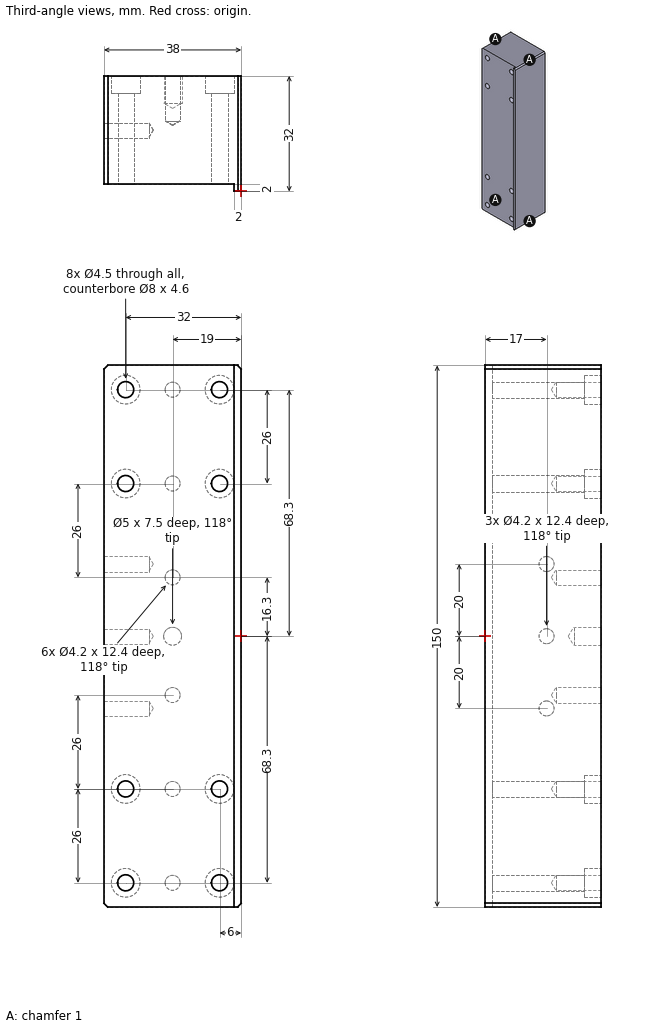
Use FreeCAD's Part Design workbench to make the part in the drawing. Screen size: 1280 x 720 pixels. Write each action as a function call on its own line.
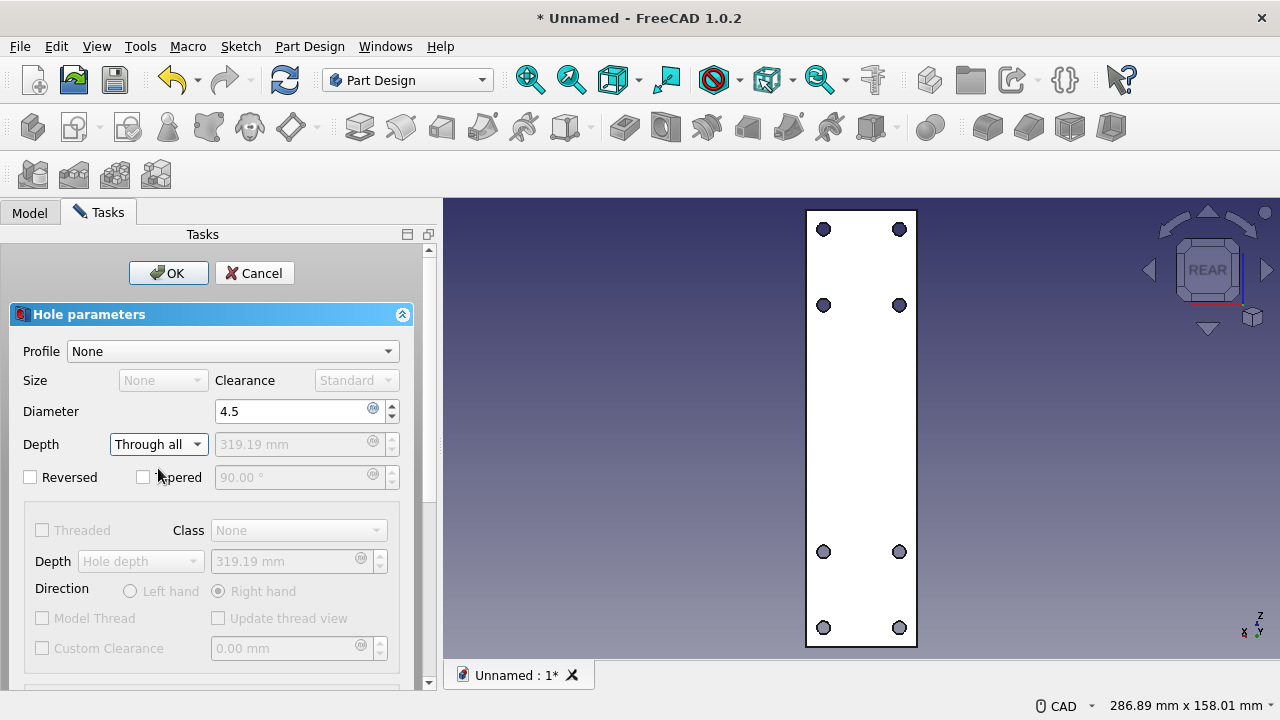
scroll(429, 467, down, 2)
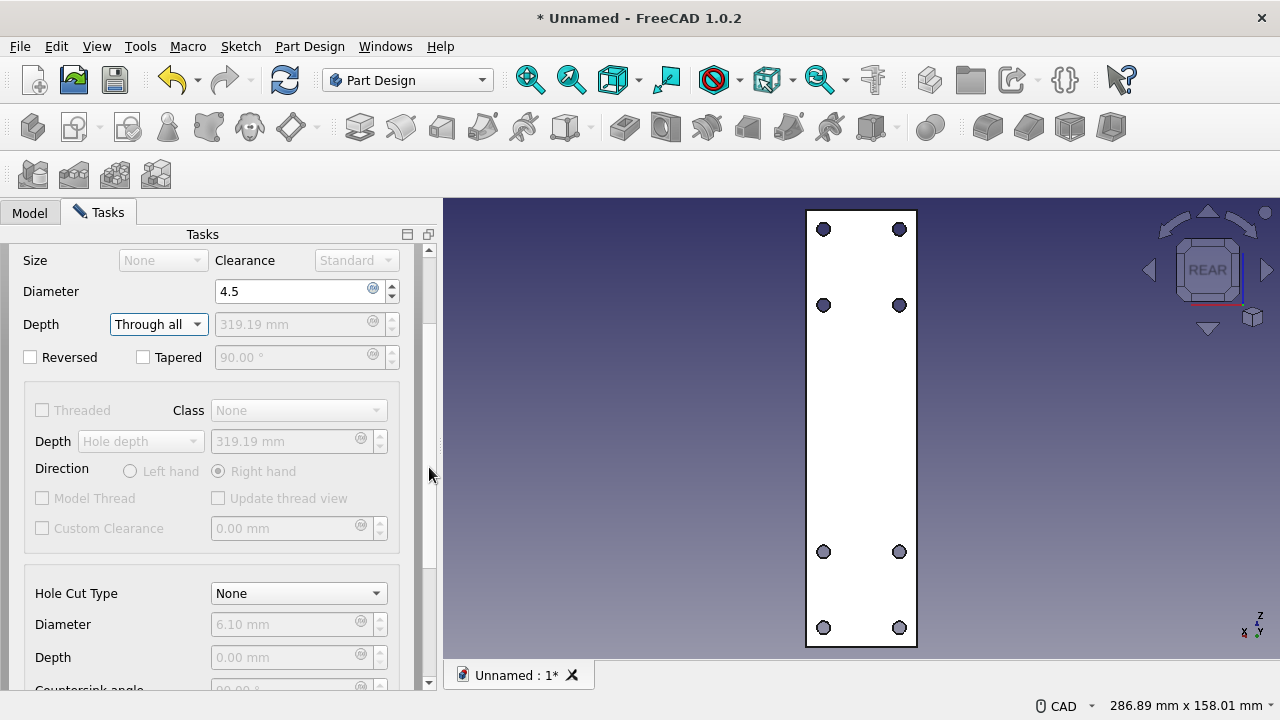
click(300, 594)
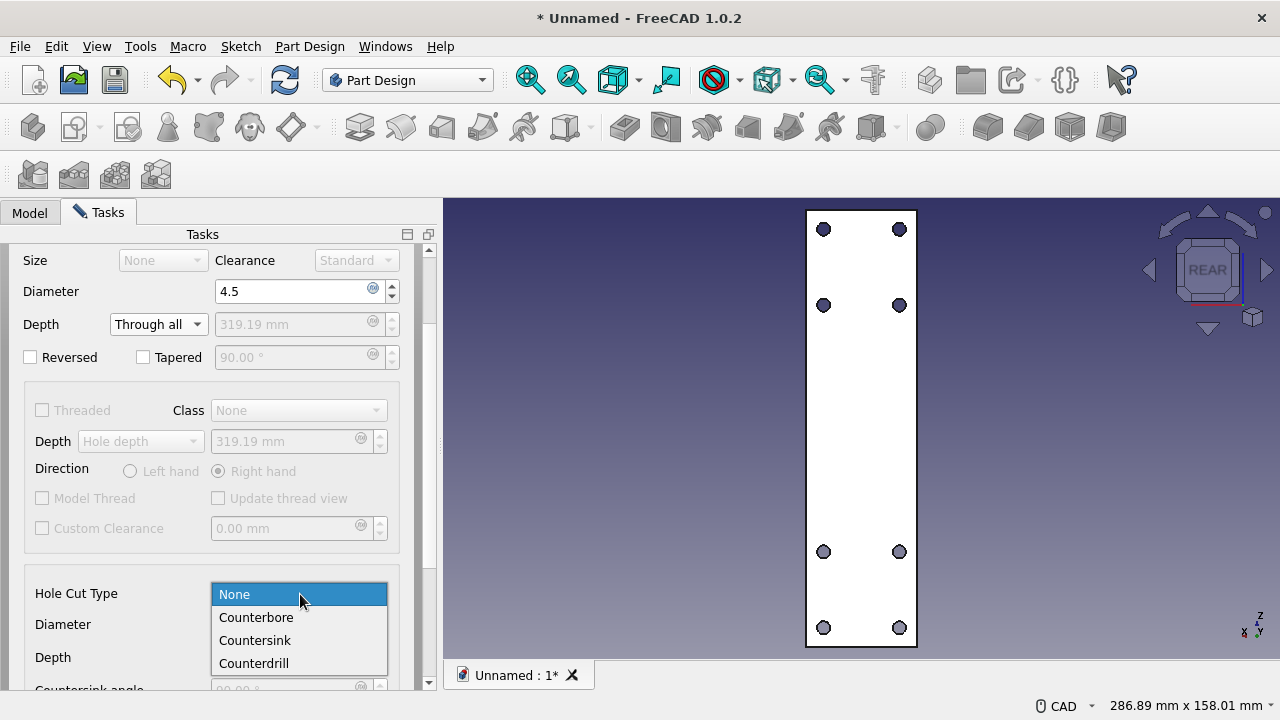
click(298, 618)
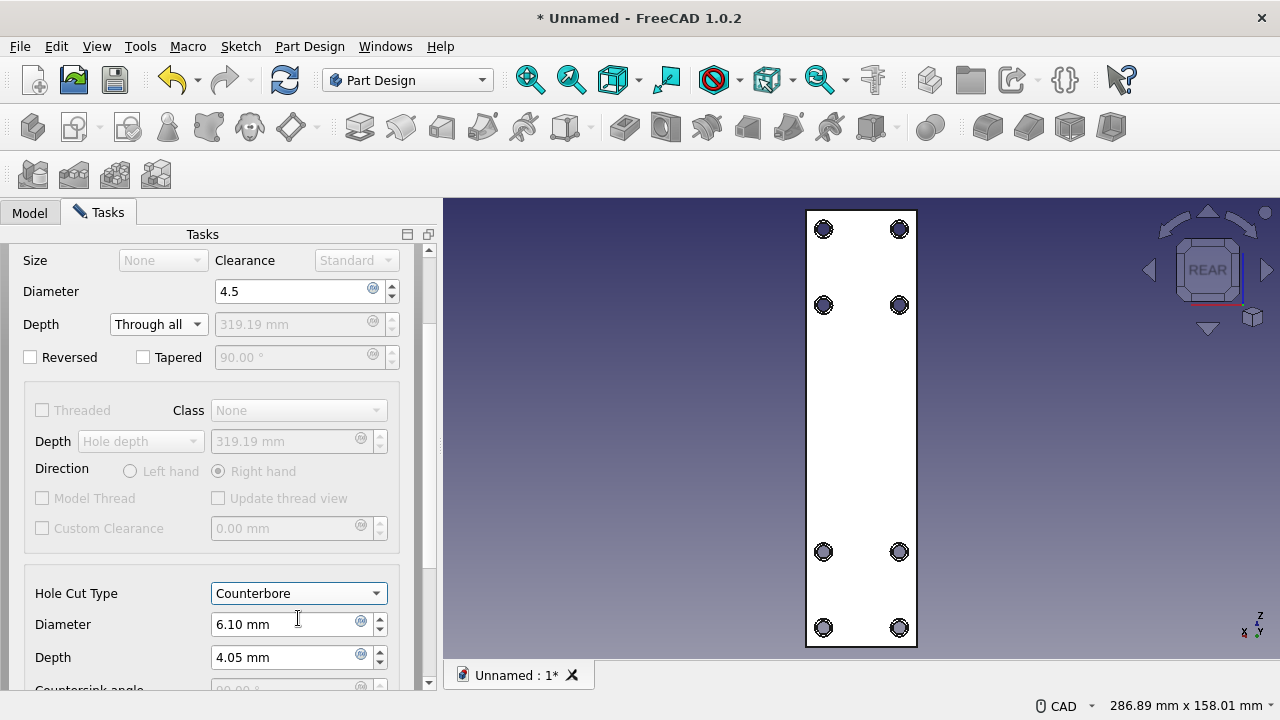
triple_click(292, 624)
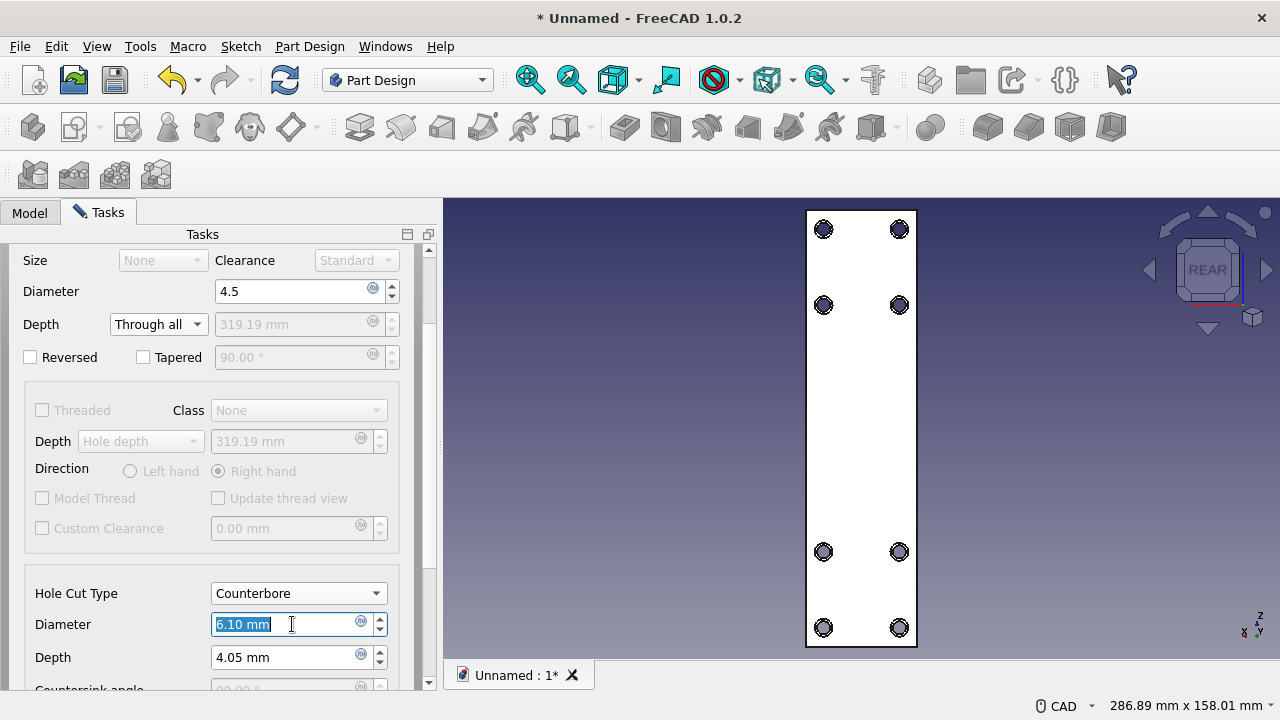
text(8)
key(Tab)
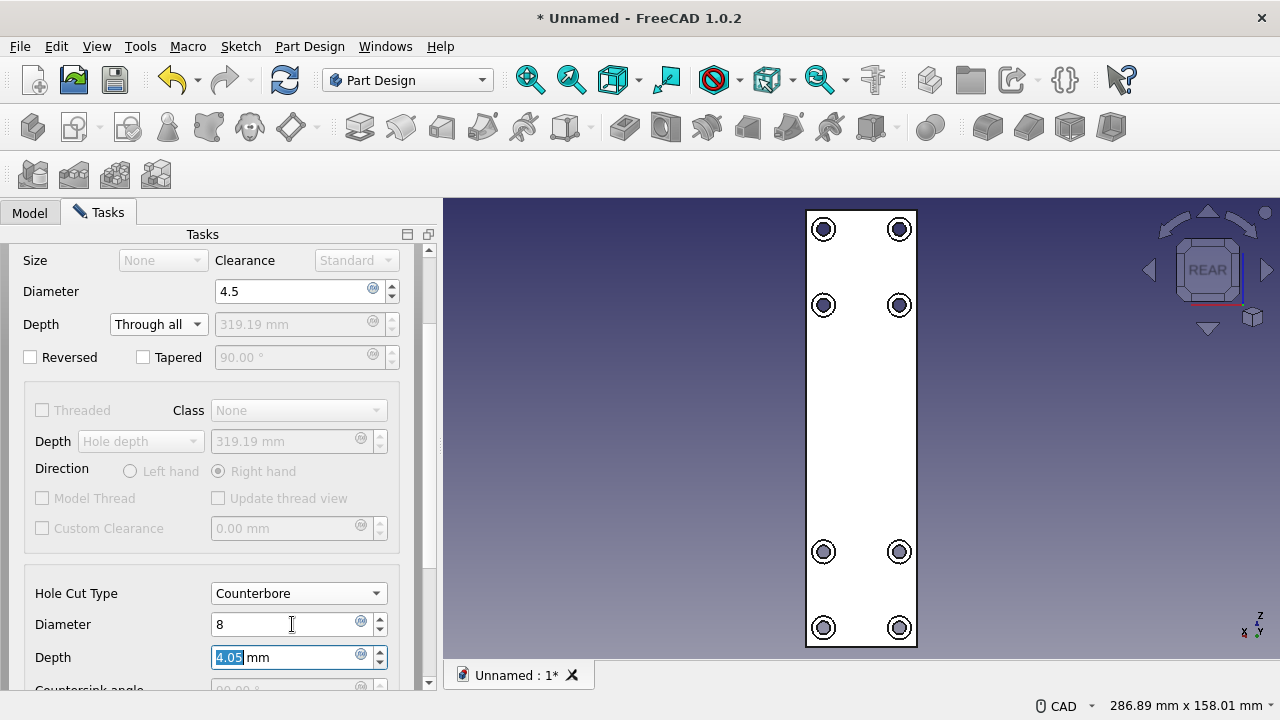
text(4.6)
key(Tab)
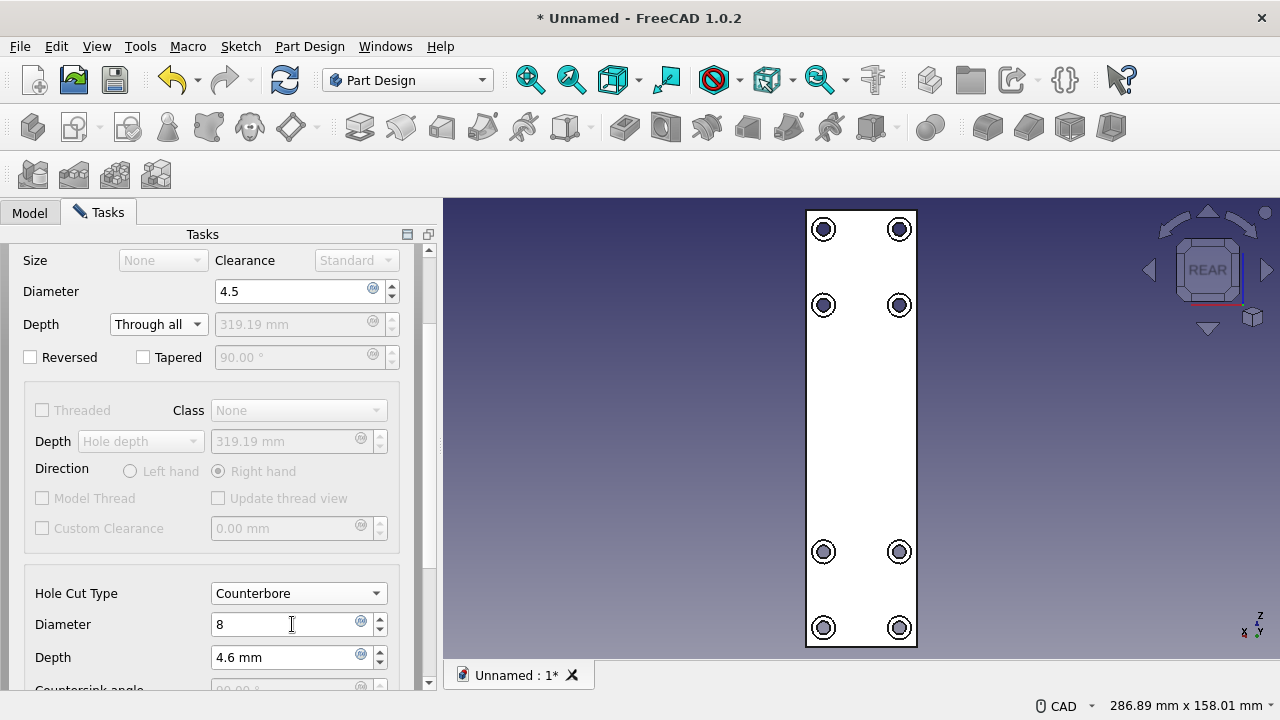
scroll(429, 467, up, 3)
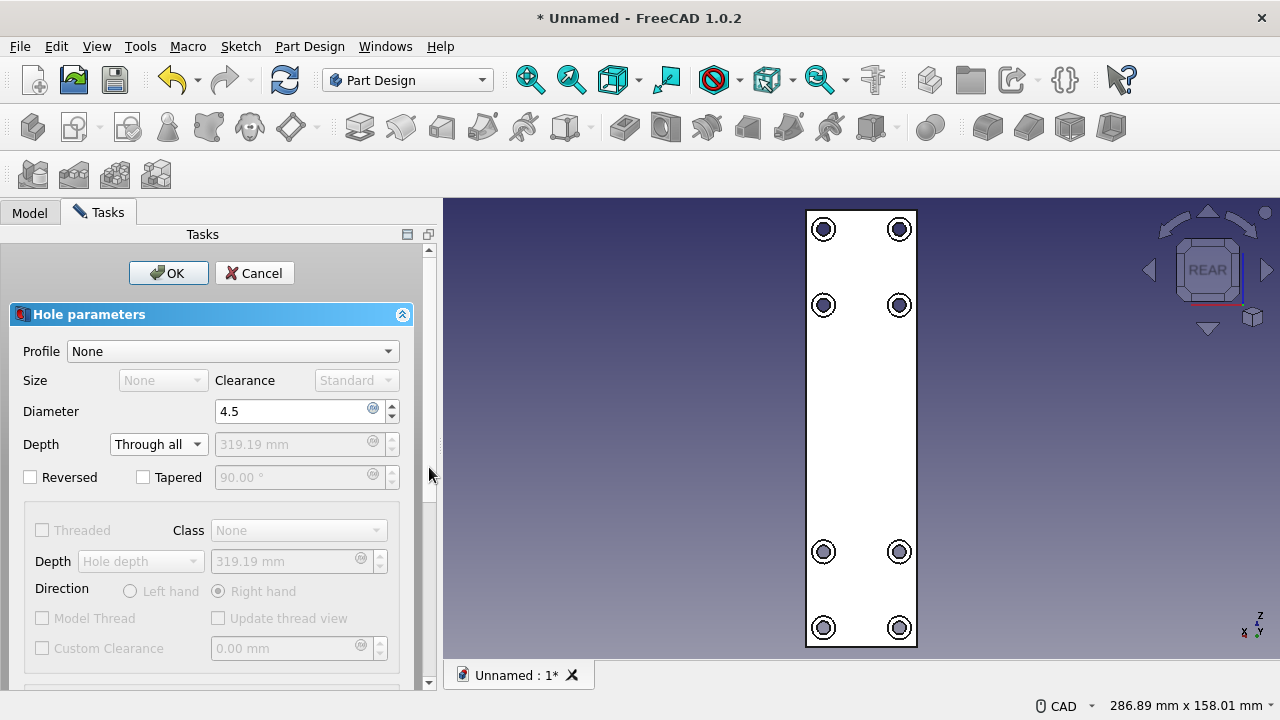
click(169, 273)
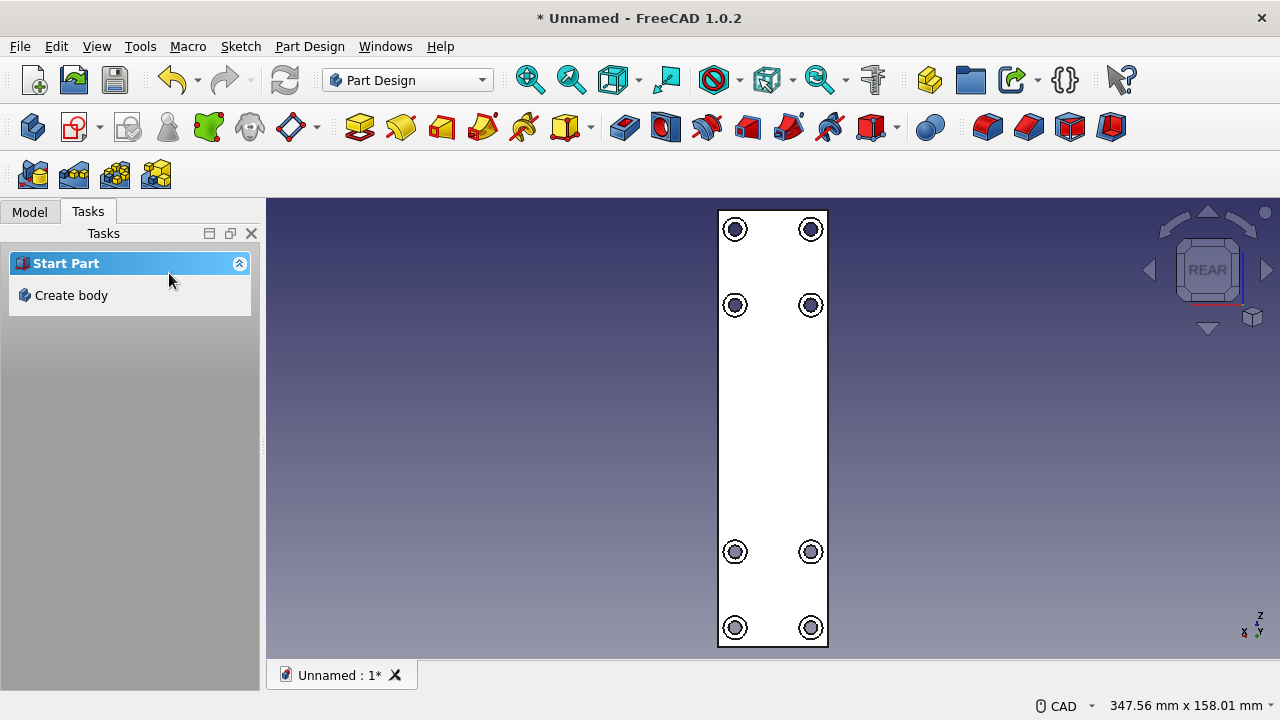
key(6)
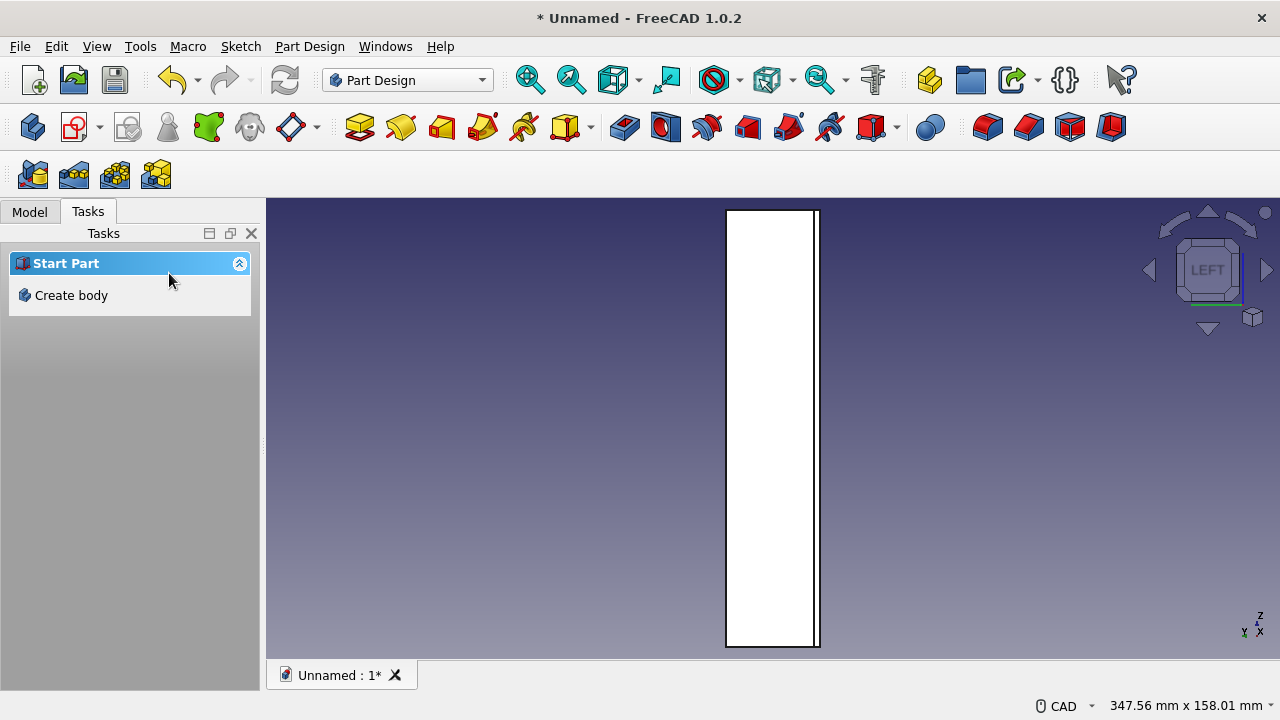
click(770, 302)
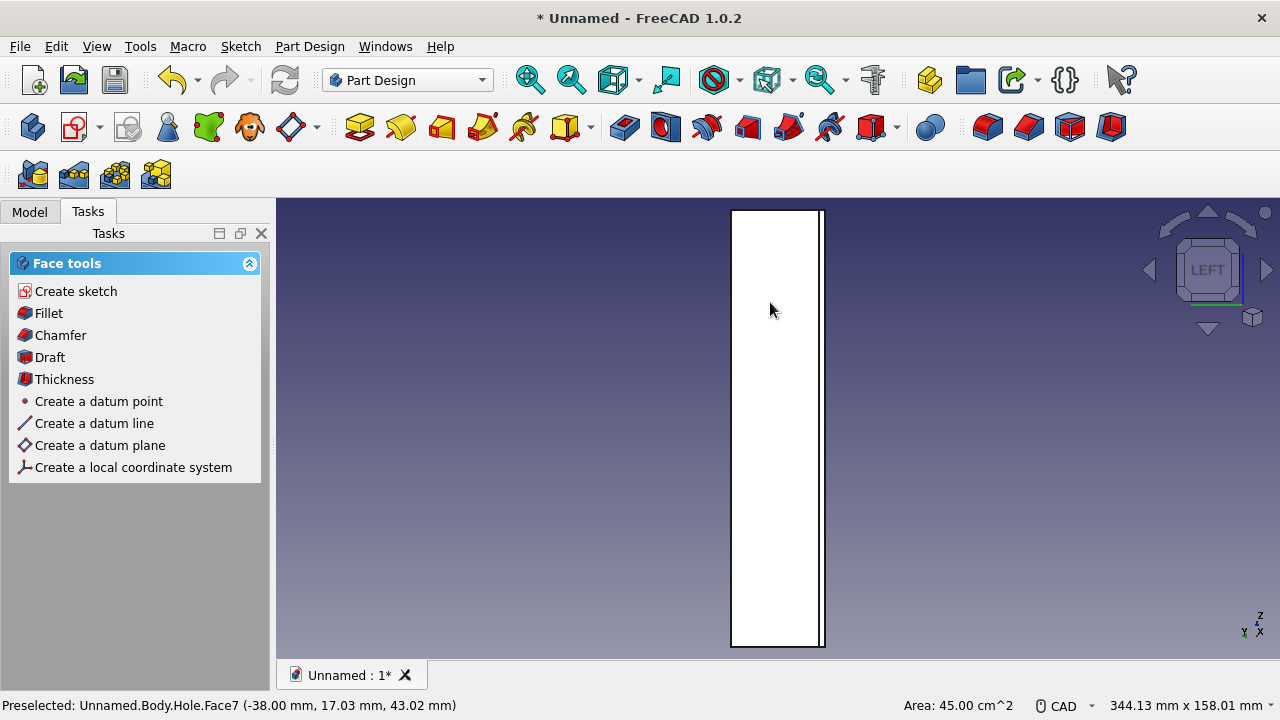
click(74, 128)